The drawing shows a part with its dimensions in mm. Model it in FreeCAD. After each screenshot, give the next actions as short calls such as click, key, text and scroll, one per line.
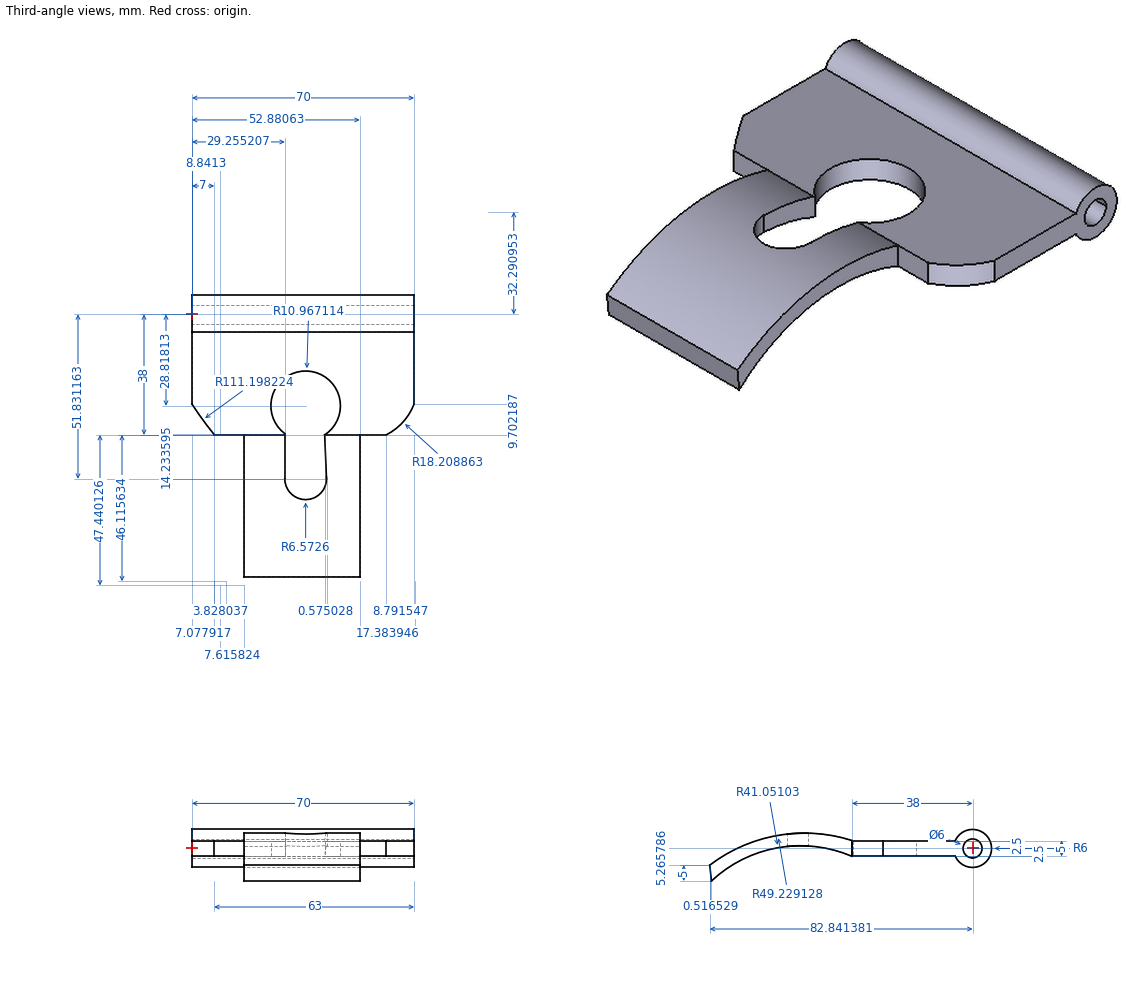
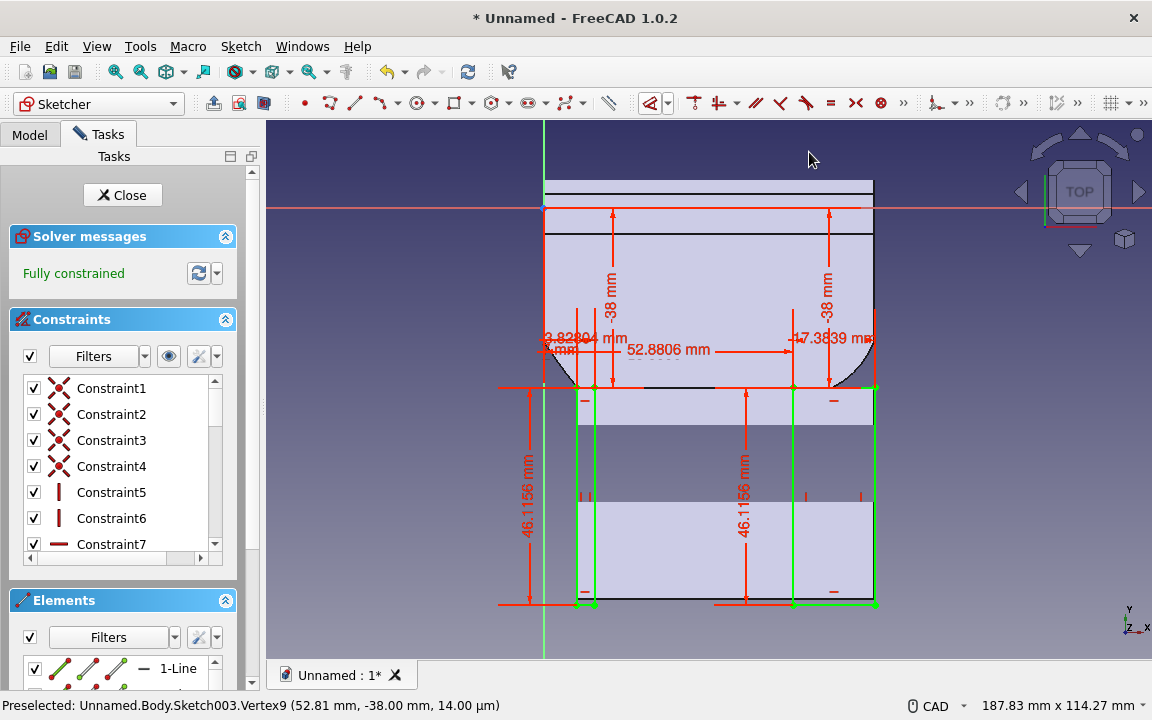
click(123, 195)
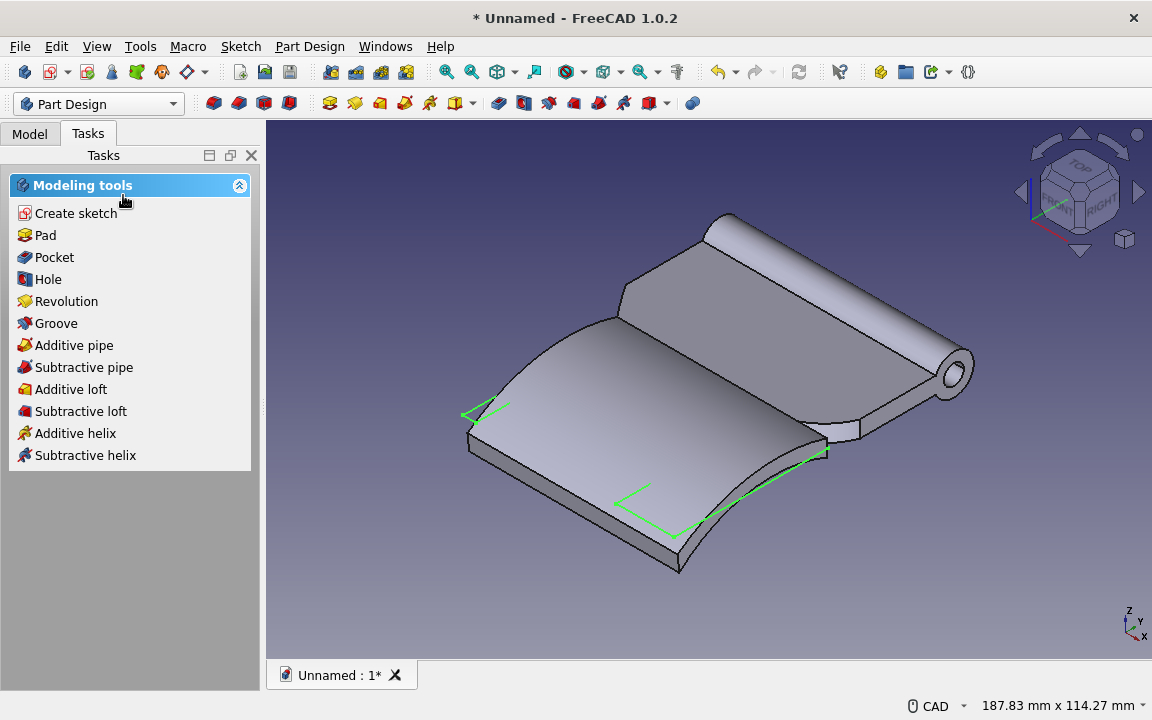
click(499, 104)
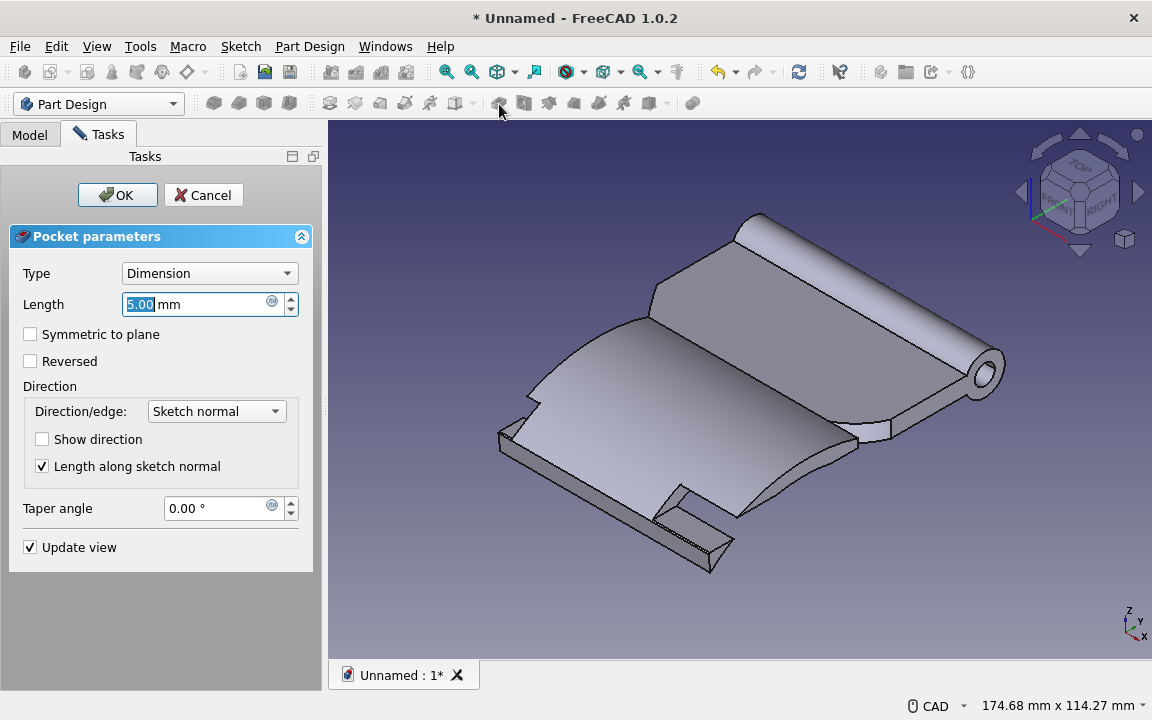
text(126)
key(Tab)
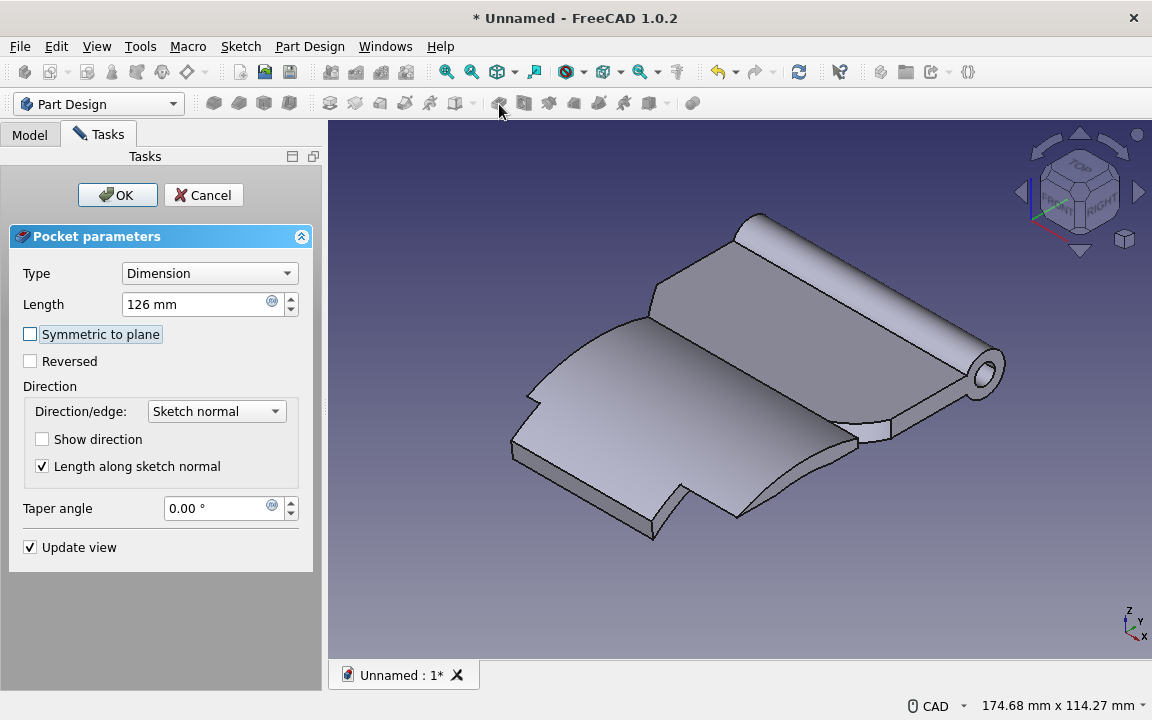
click(31, 334)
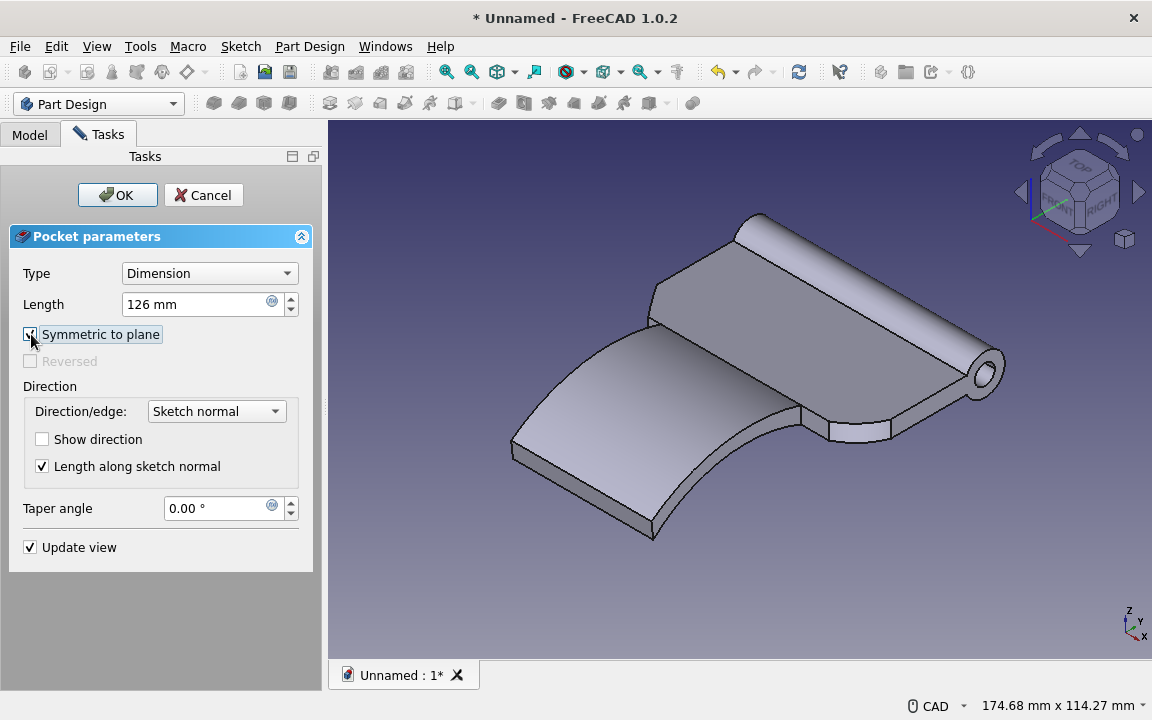
click(118, 195)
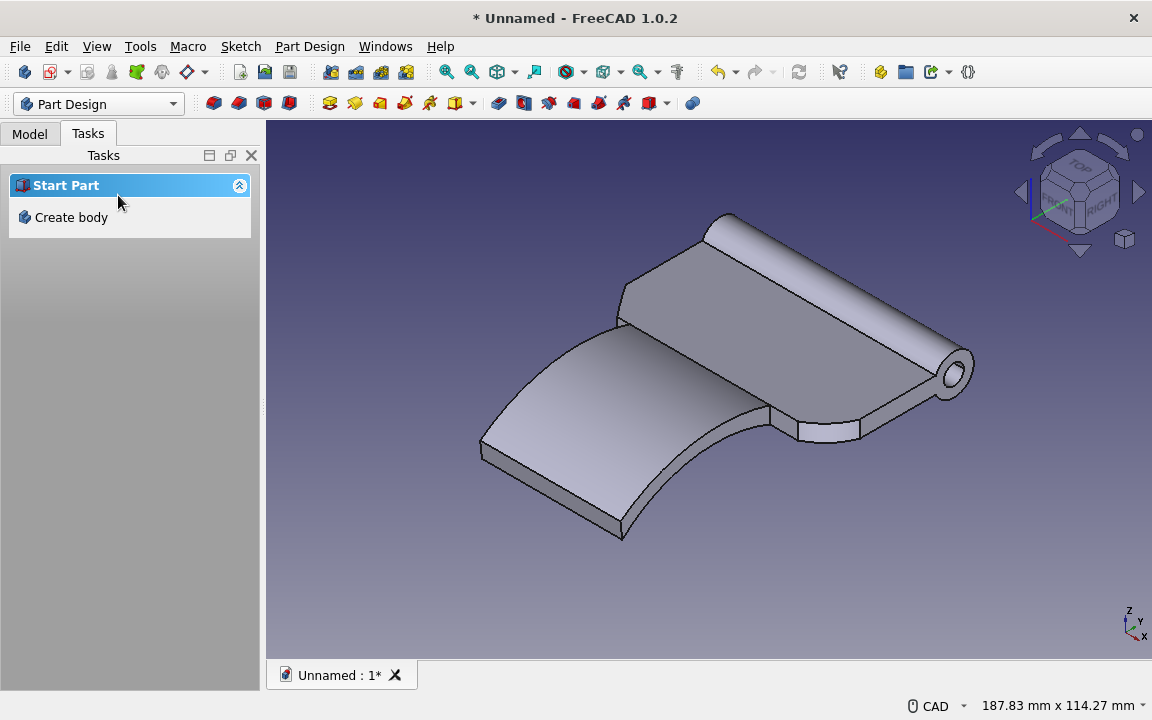
click(50, 72)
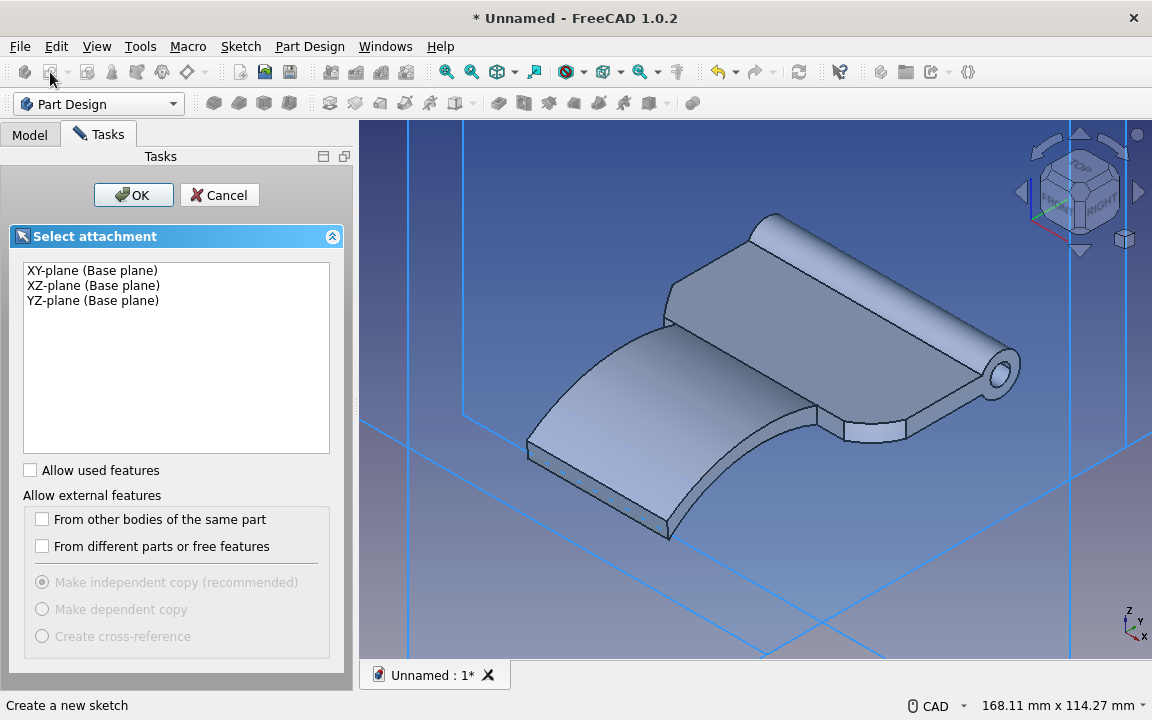
click(84, 270)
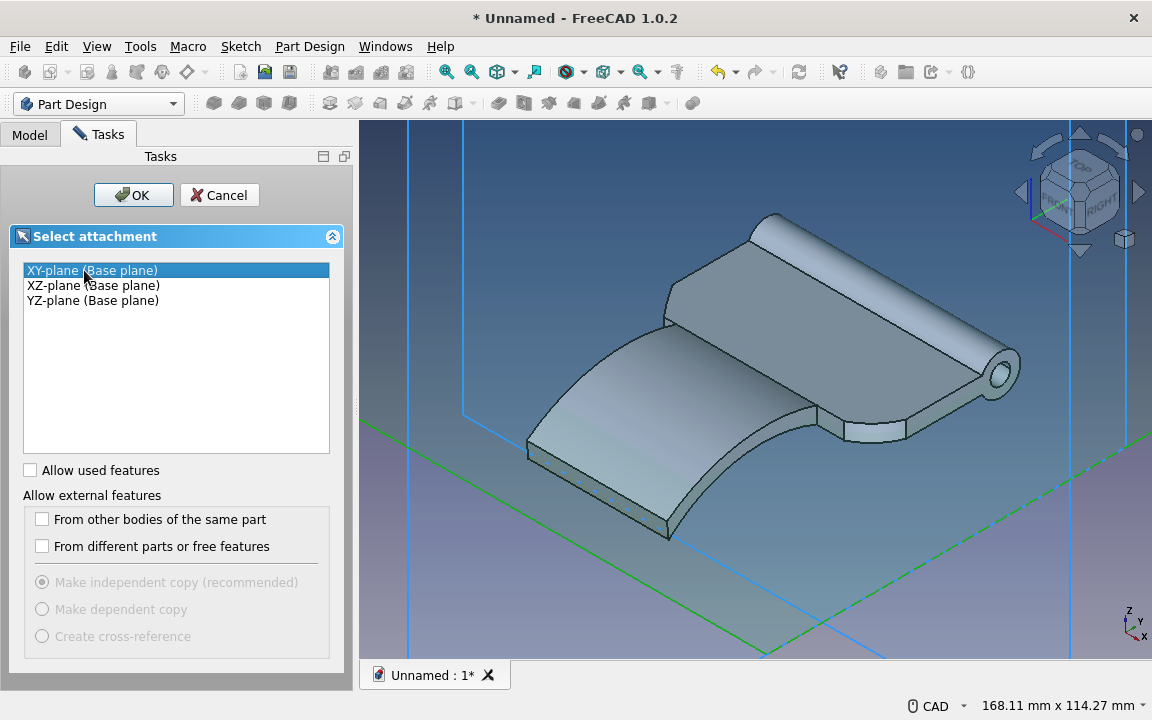
click(134, 195)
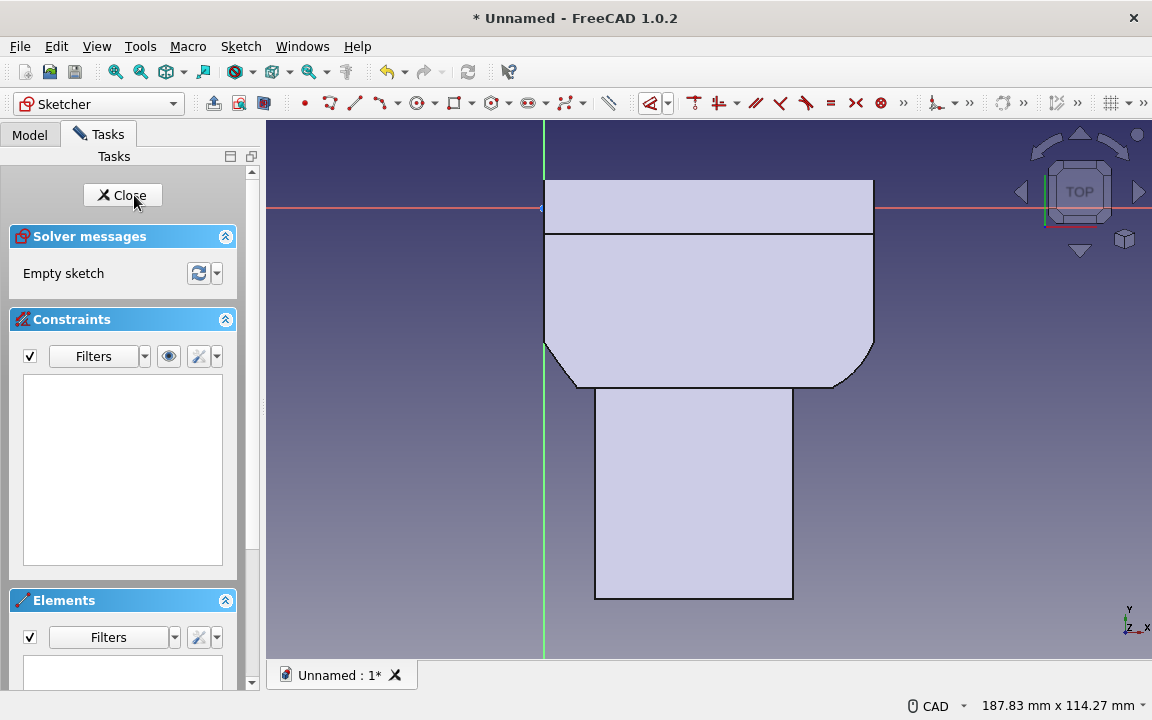
click(264, 104)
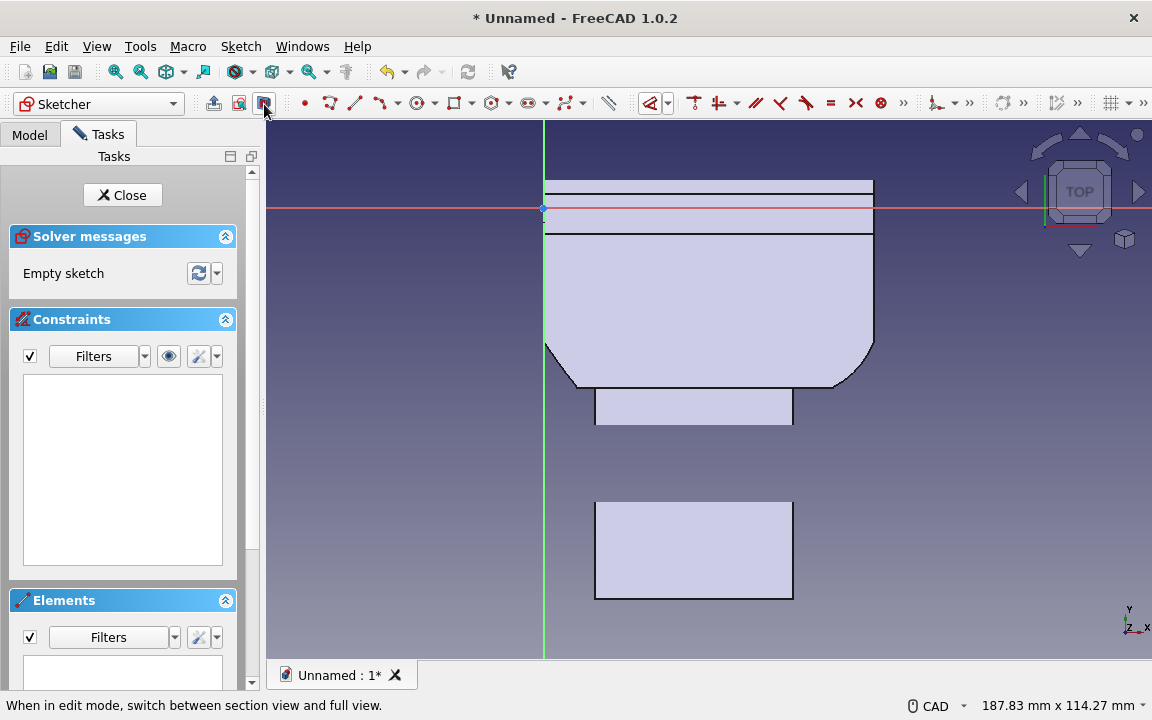
scroll(901, 298, down, 1)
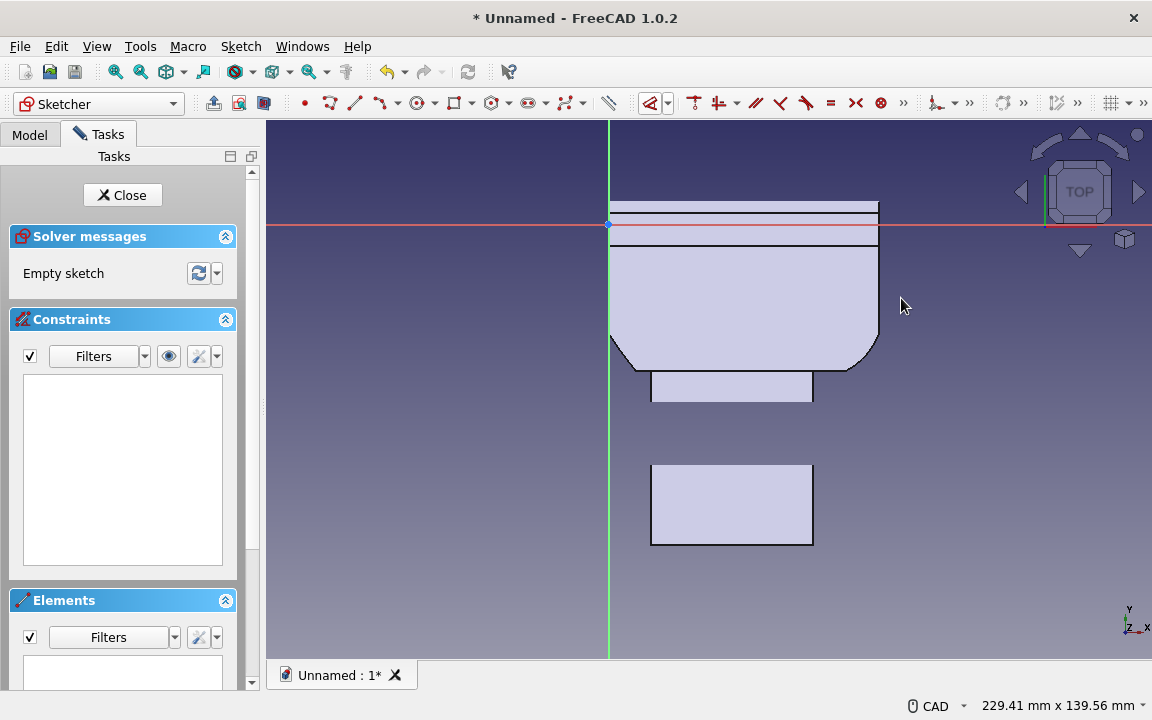
click(454, 104)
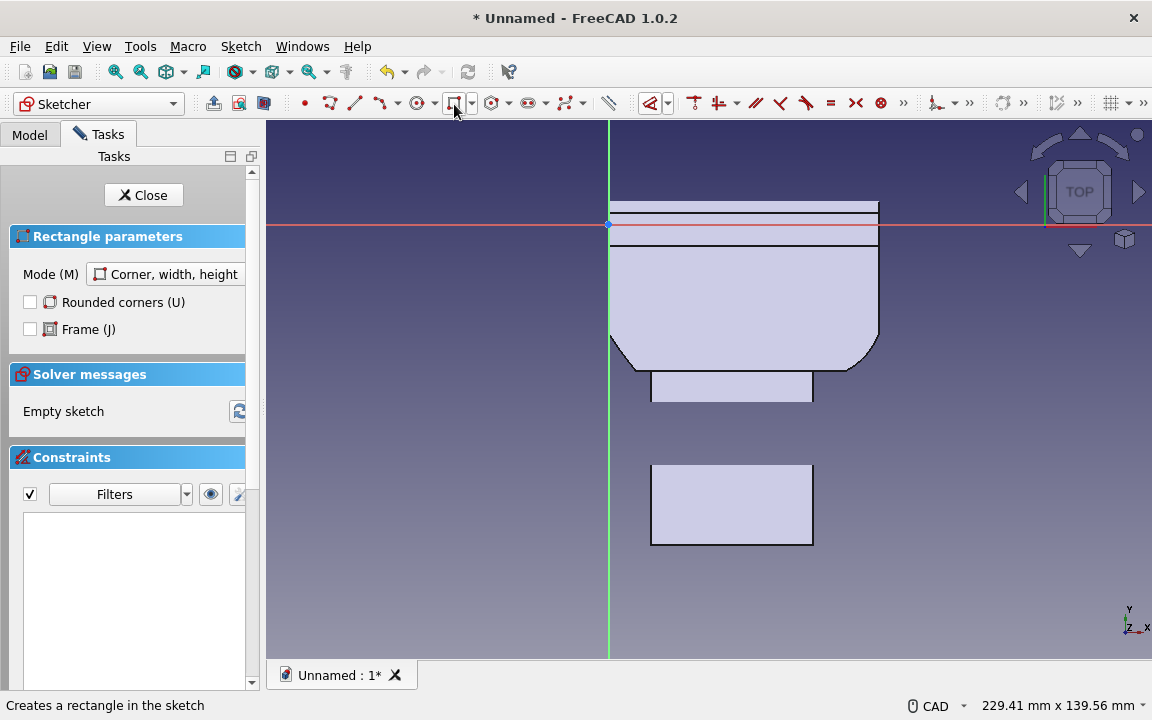
click(643, 371)
move(672, 555)